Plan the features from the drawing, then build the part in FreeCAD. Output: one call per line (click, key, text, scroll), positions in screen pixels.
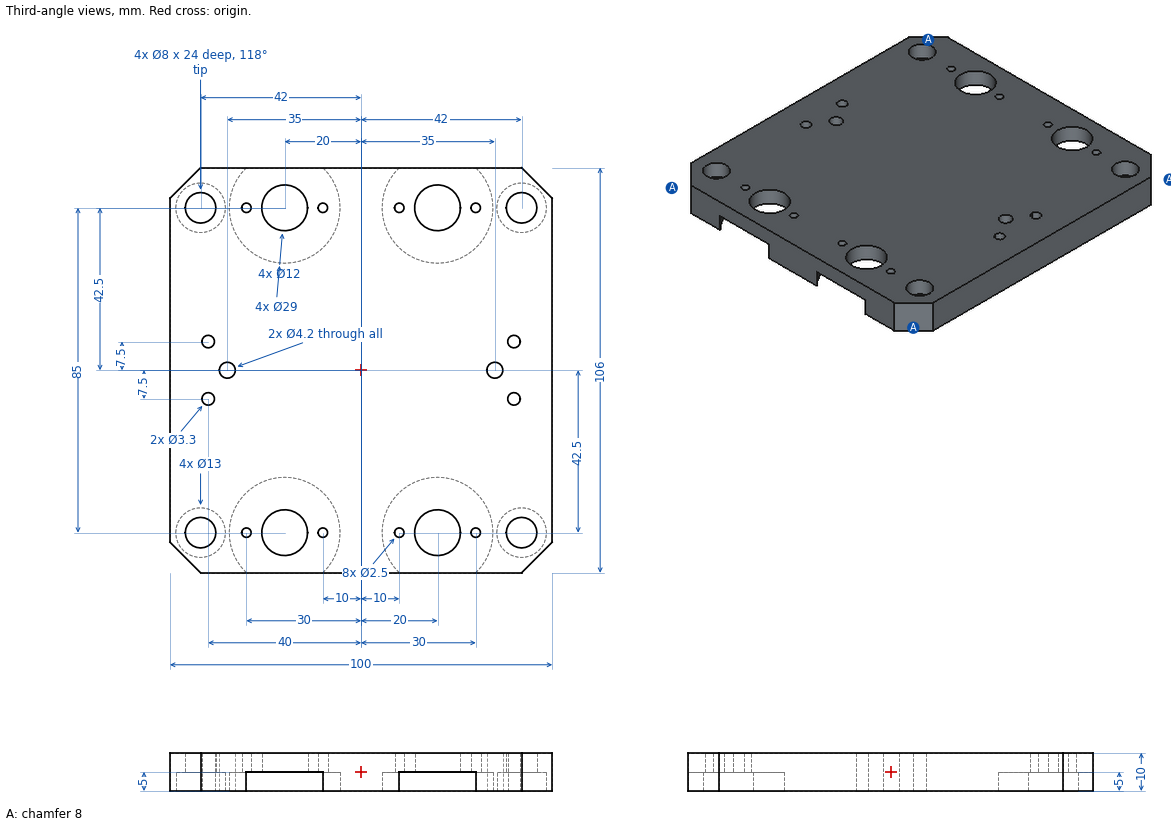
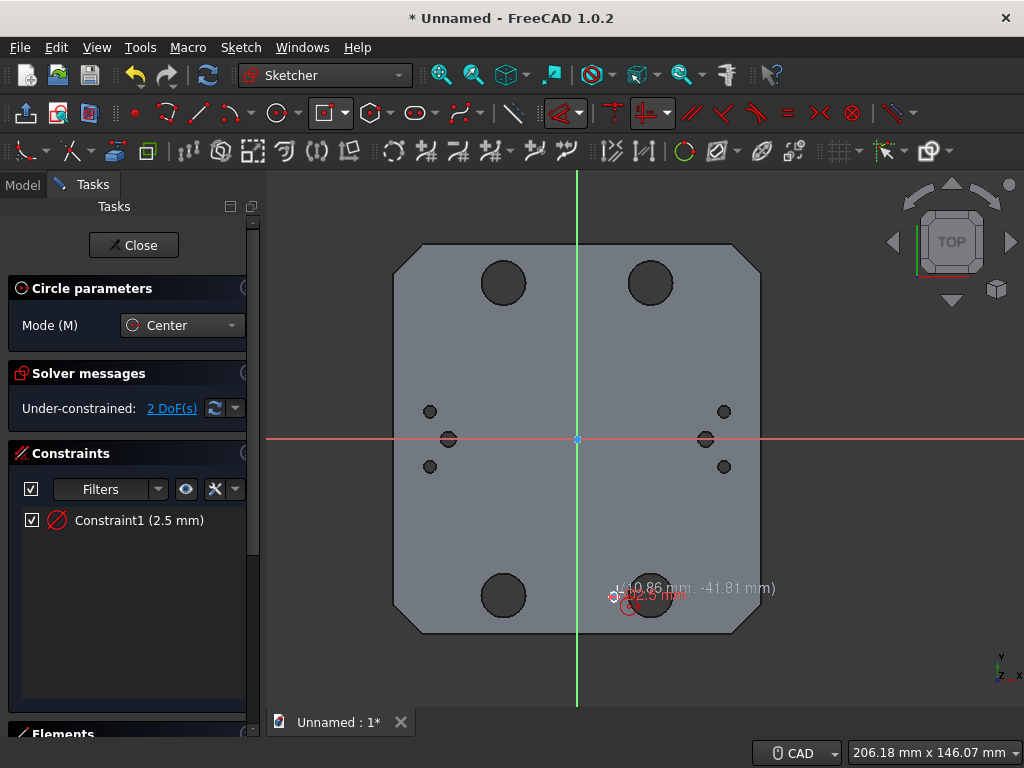
scroll(687, 596, up, 8)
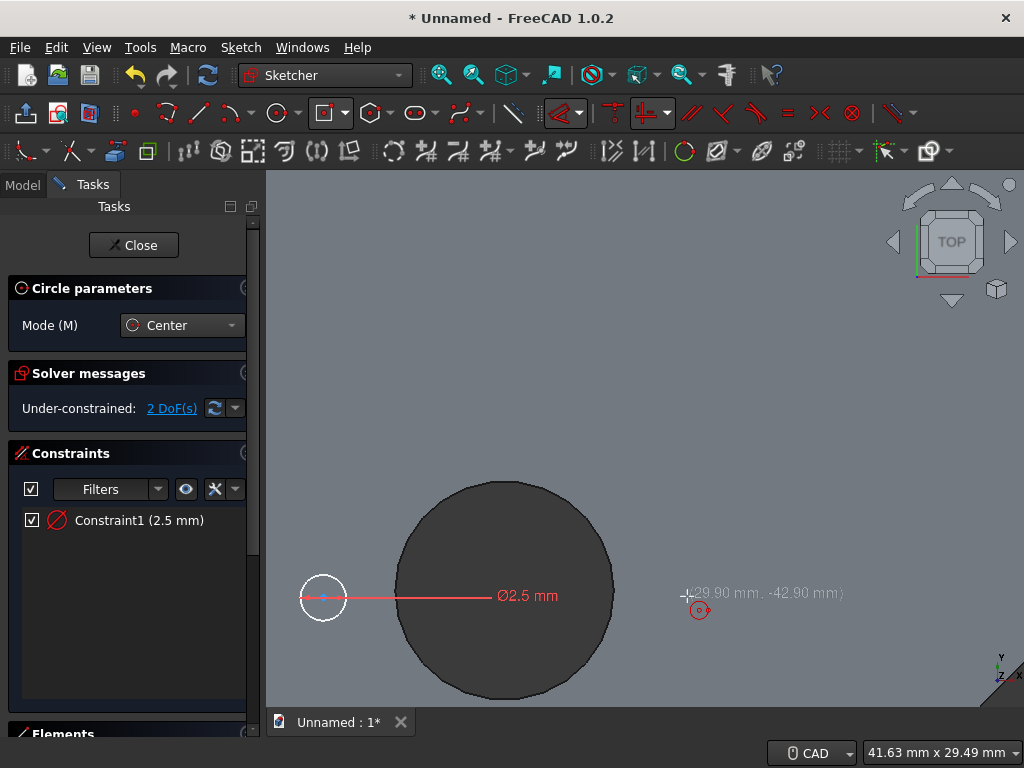
scroll(687, 596, down, 8)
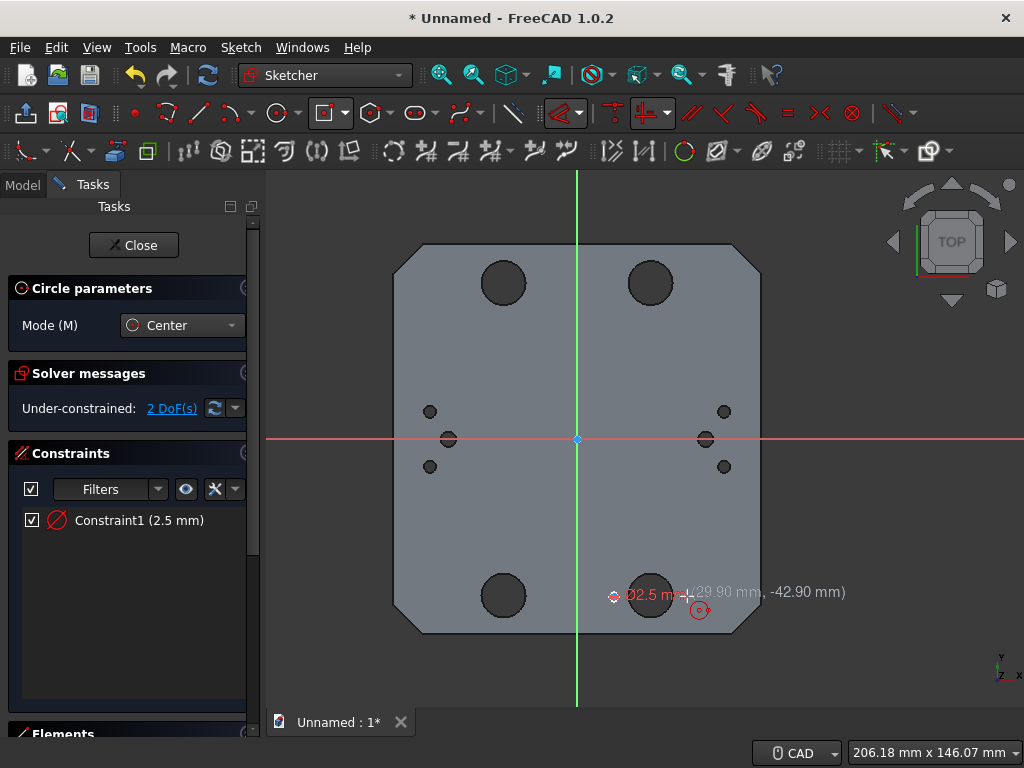
click(687, 596)
move(691, 592)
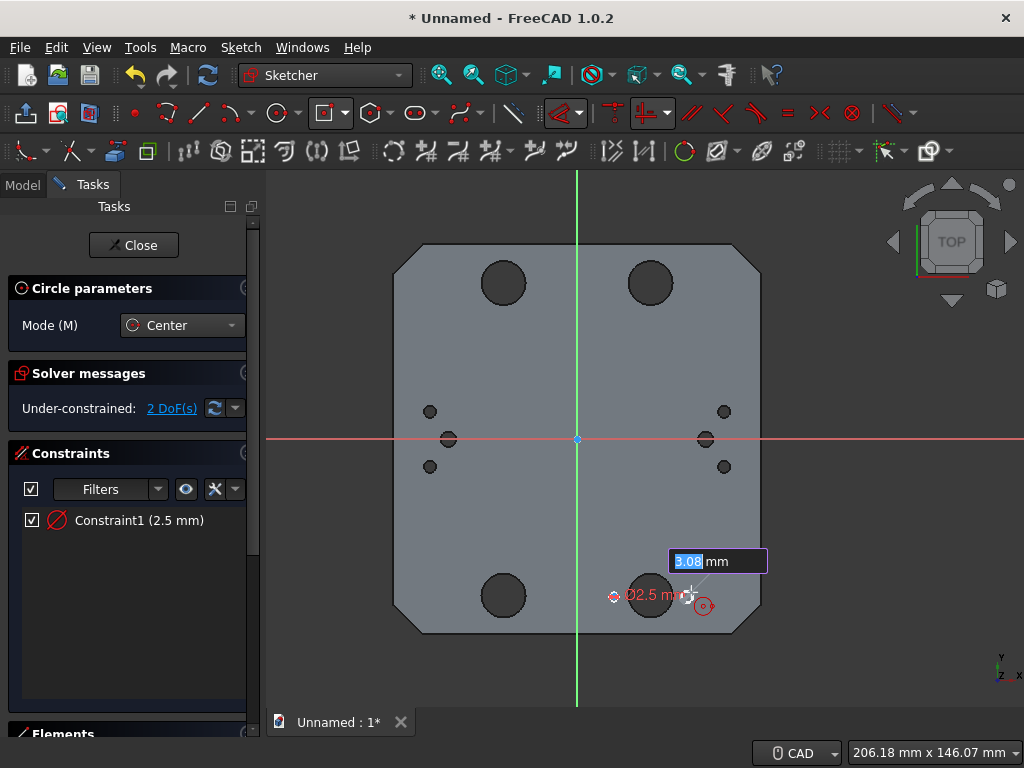
text(2.5)
key(Return)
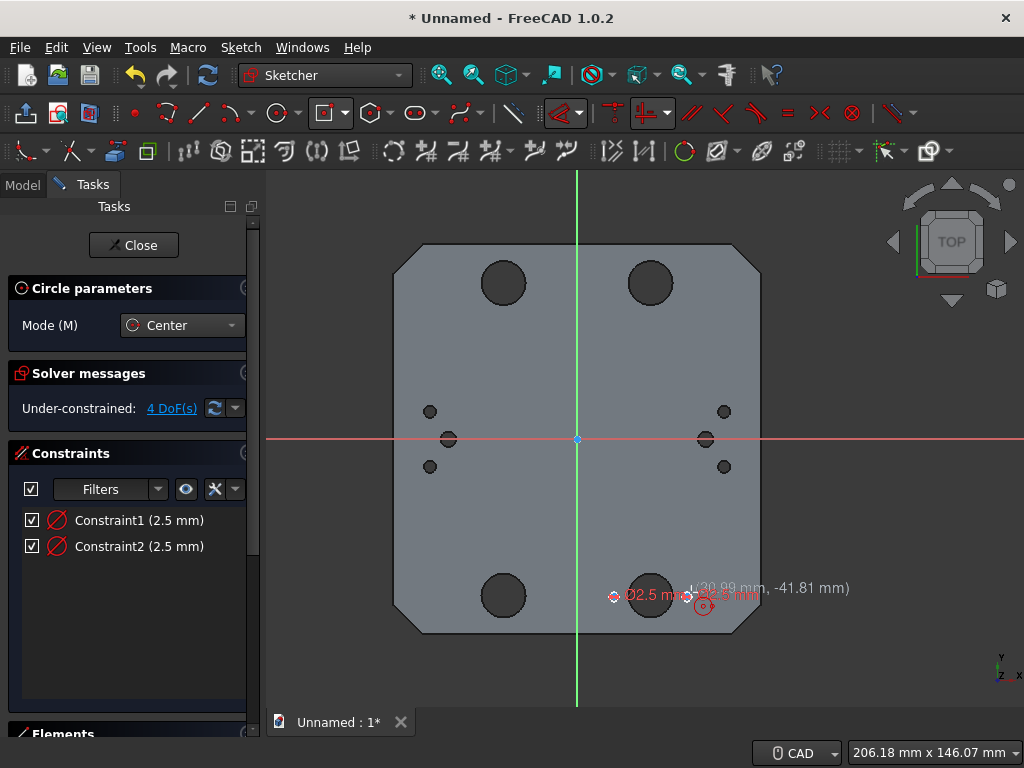
scroll(540, 596, up, 8)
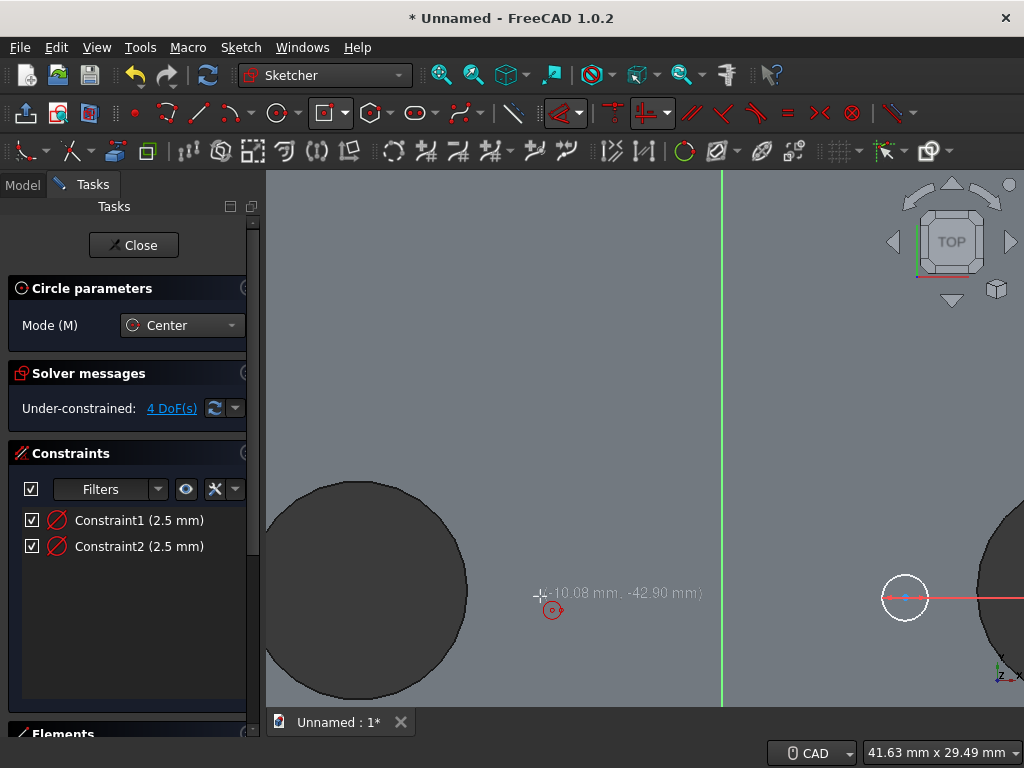
scroll(540, 596, down, 8)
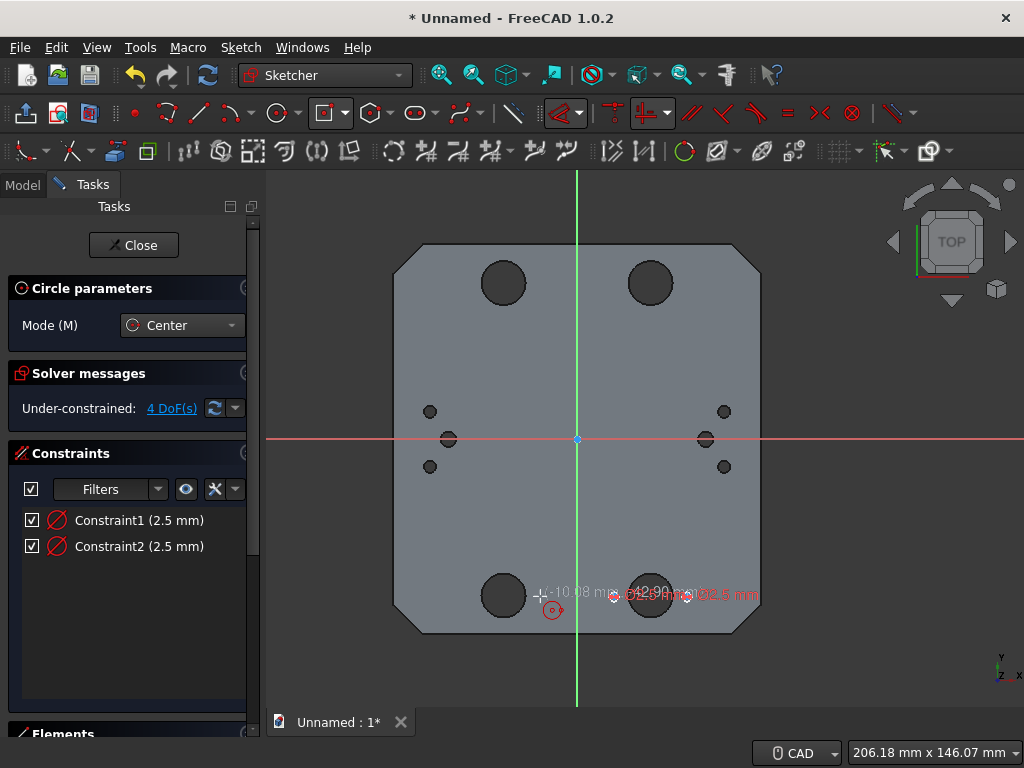
click(540, 596)
move(544, 592)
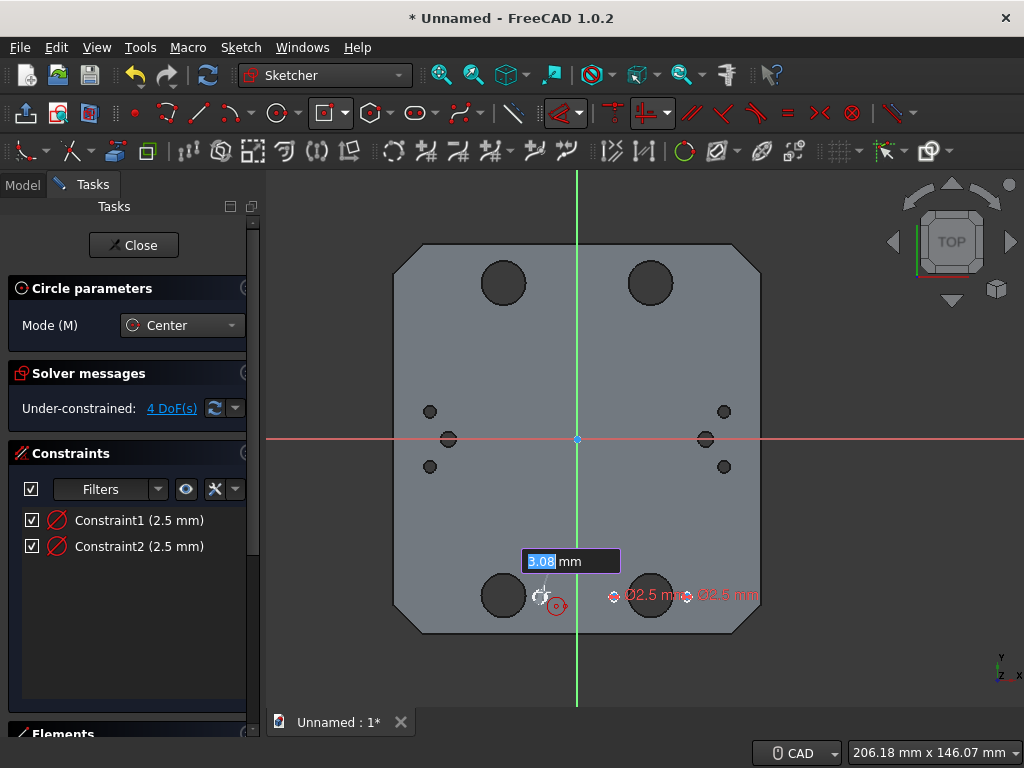
text(2.5)
key(Return)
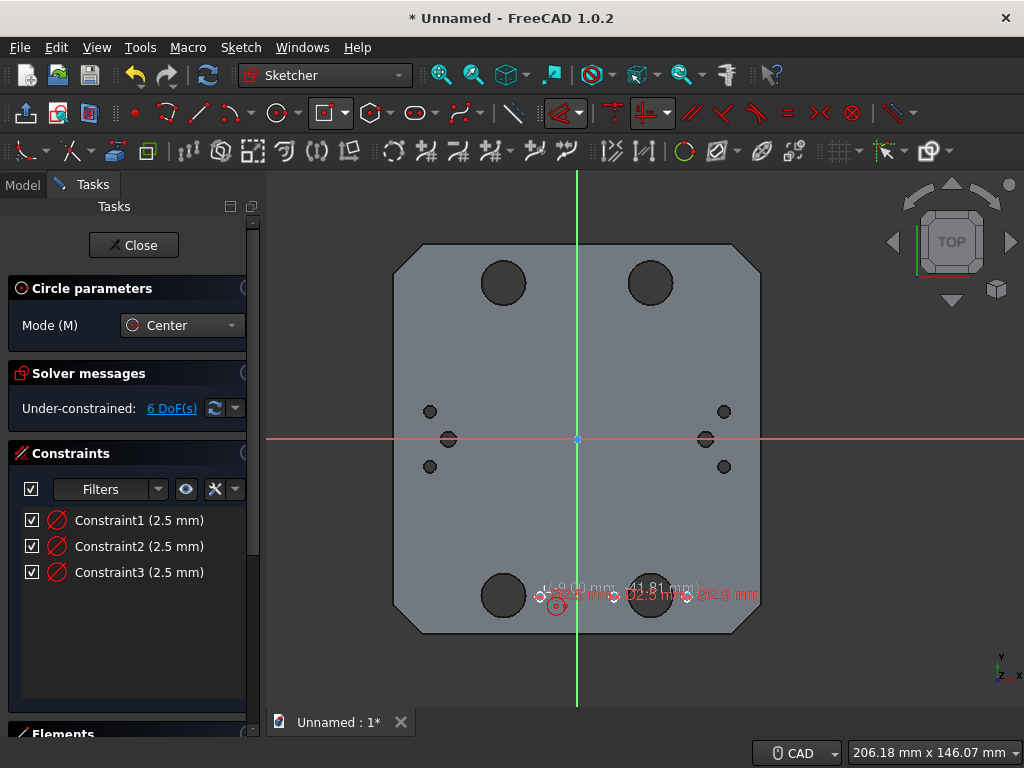
scroll(467, 596, up, 8)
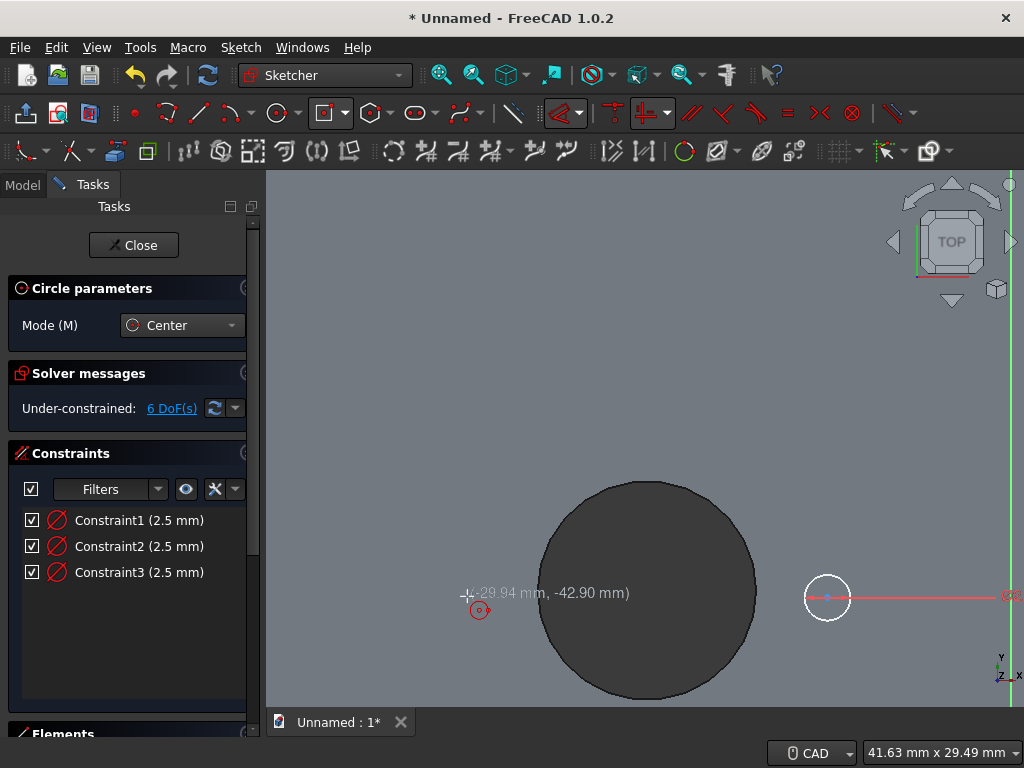
scroll(467, 596, down, 8)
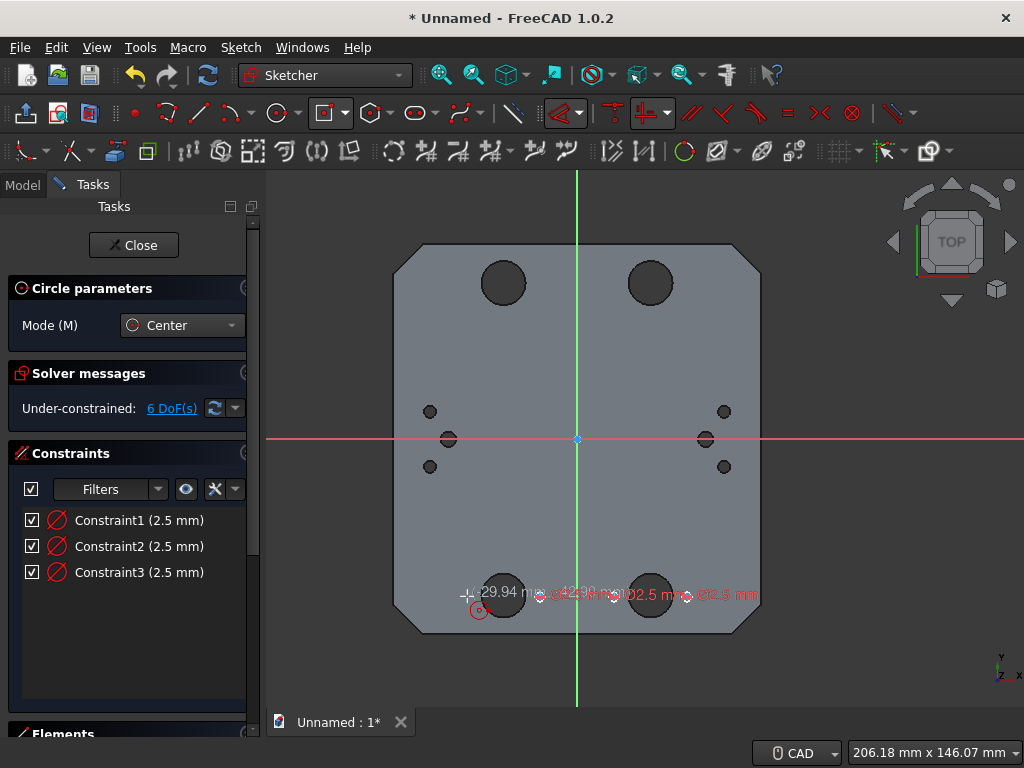
click(467, 596)
move(470, 592)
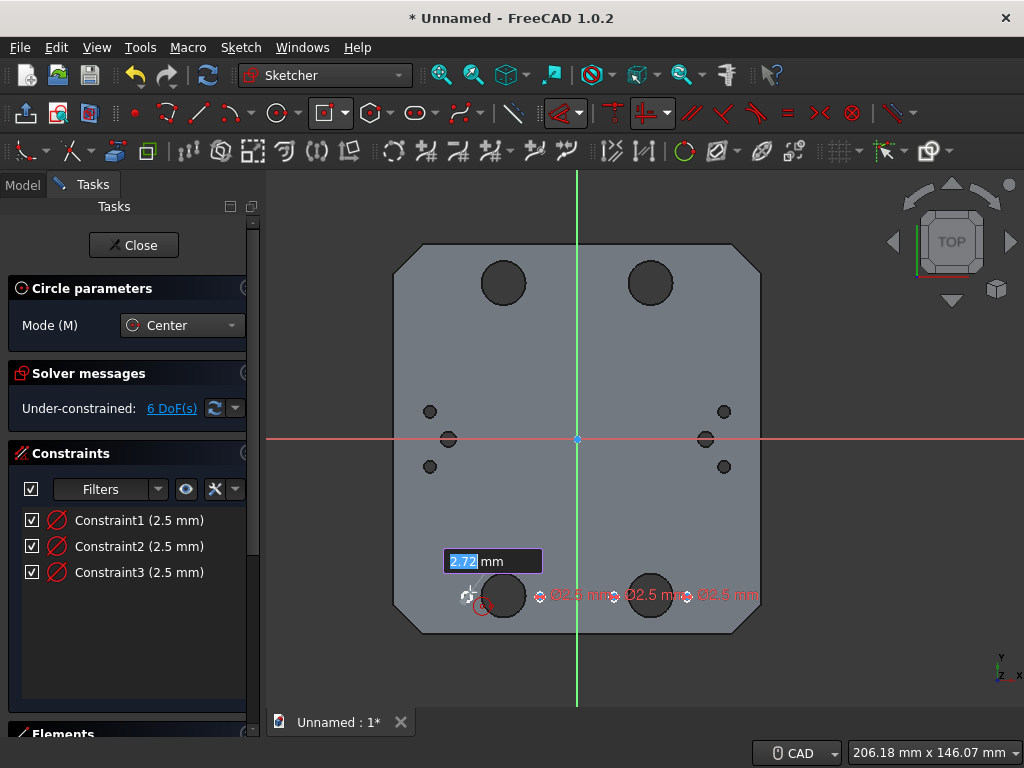
text(2.5)
key(Return)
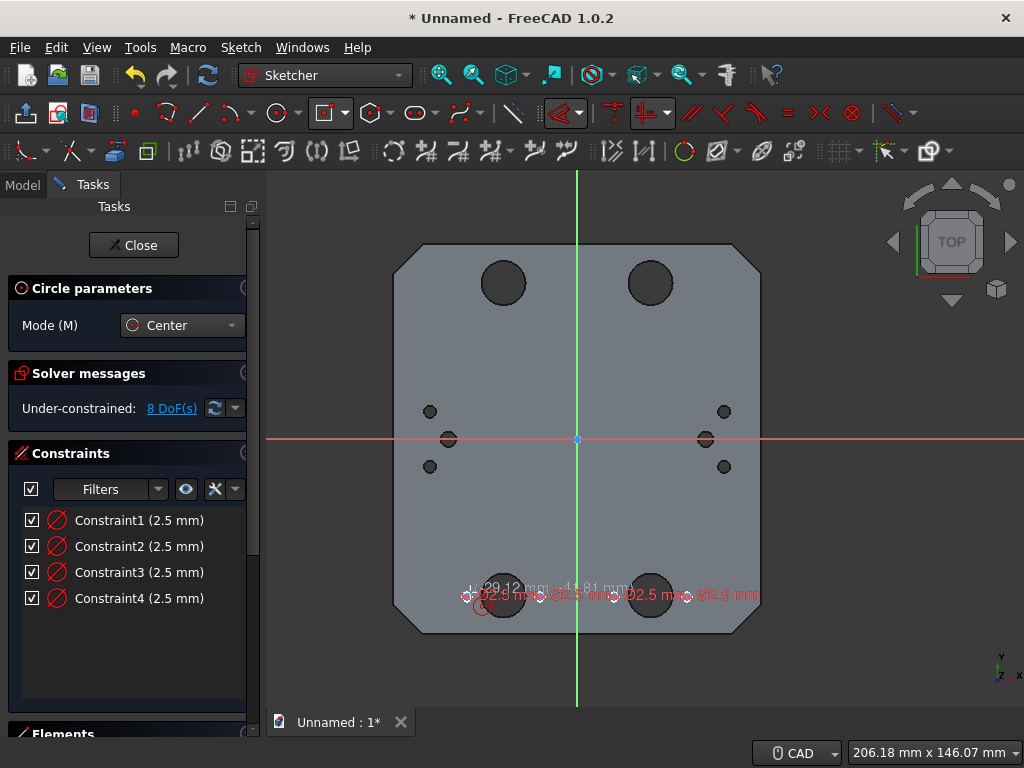
scroll(540, 283, up, 8)